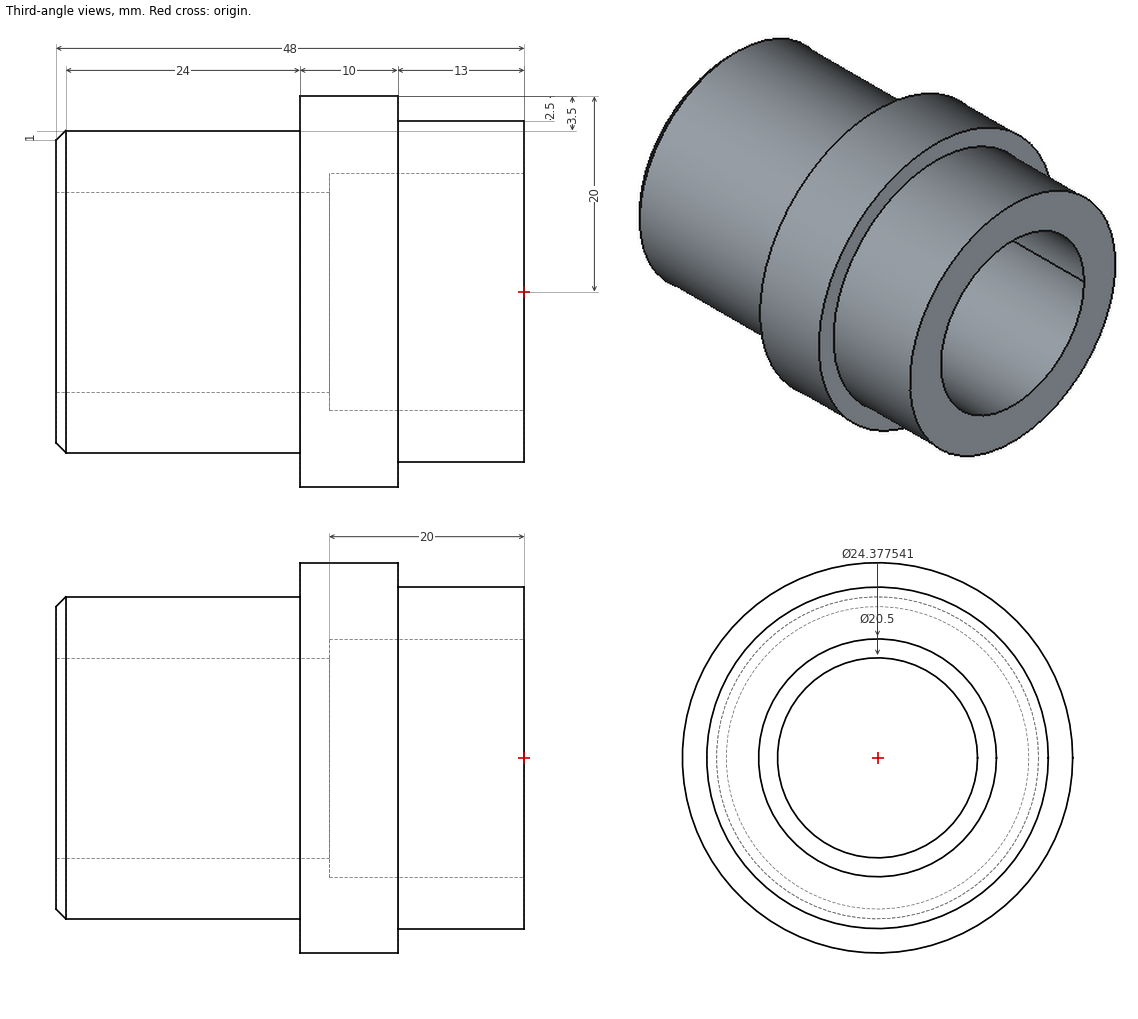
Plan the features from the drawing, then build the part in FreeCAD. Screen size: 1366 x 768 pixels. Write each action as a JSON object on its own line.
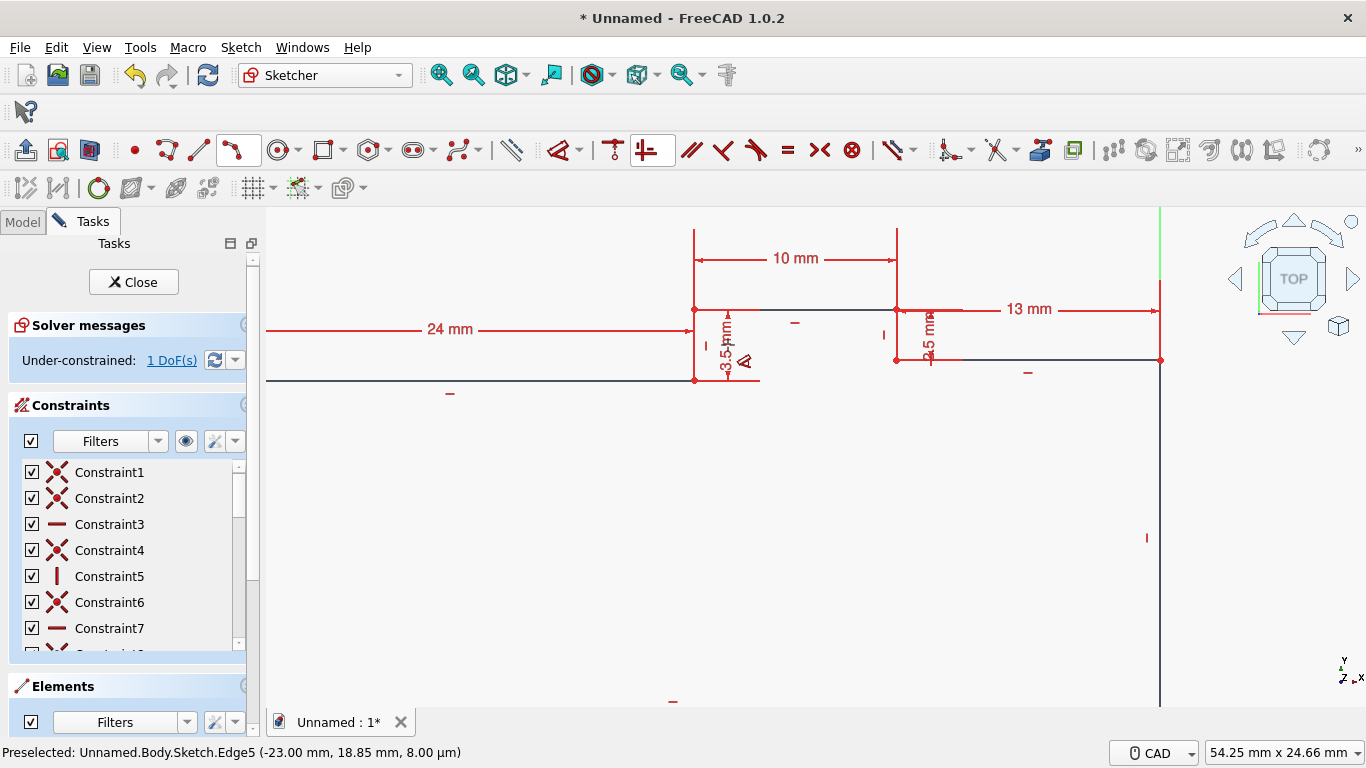
{"action": "left_click", "coordinate": [897, 310]}
{"action": "left_click", "coordinate": [1194, 494]}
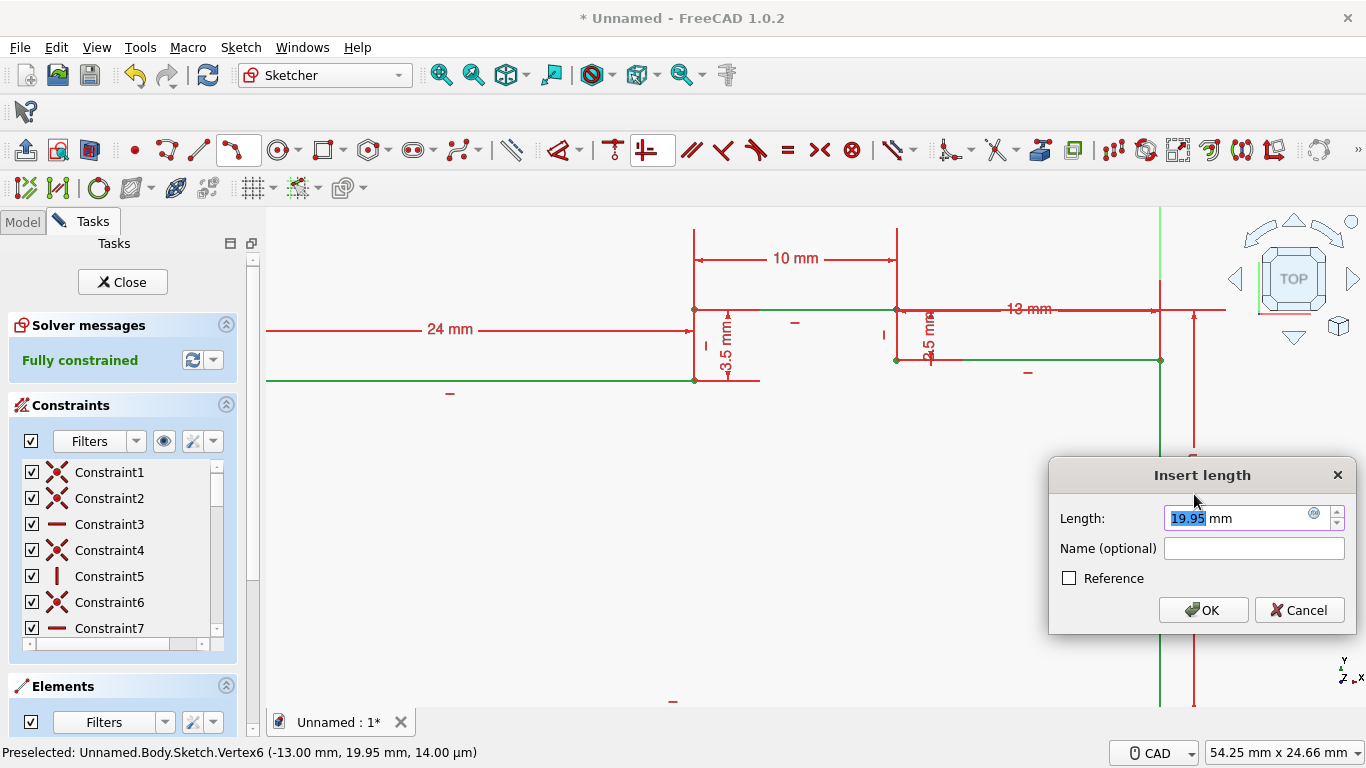
{"action": "type", "text": "20"}
{"action": "key", "text": "Return"}
{"action": "key", "text": "Escape"}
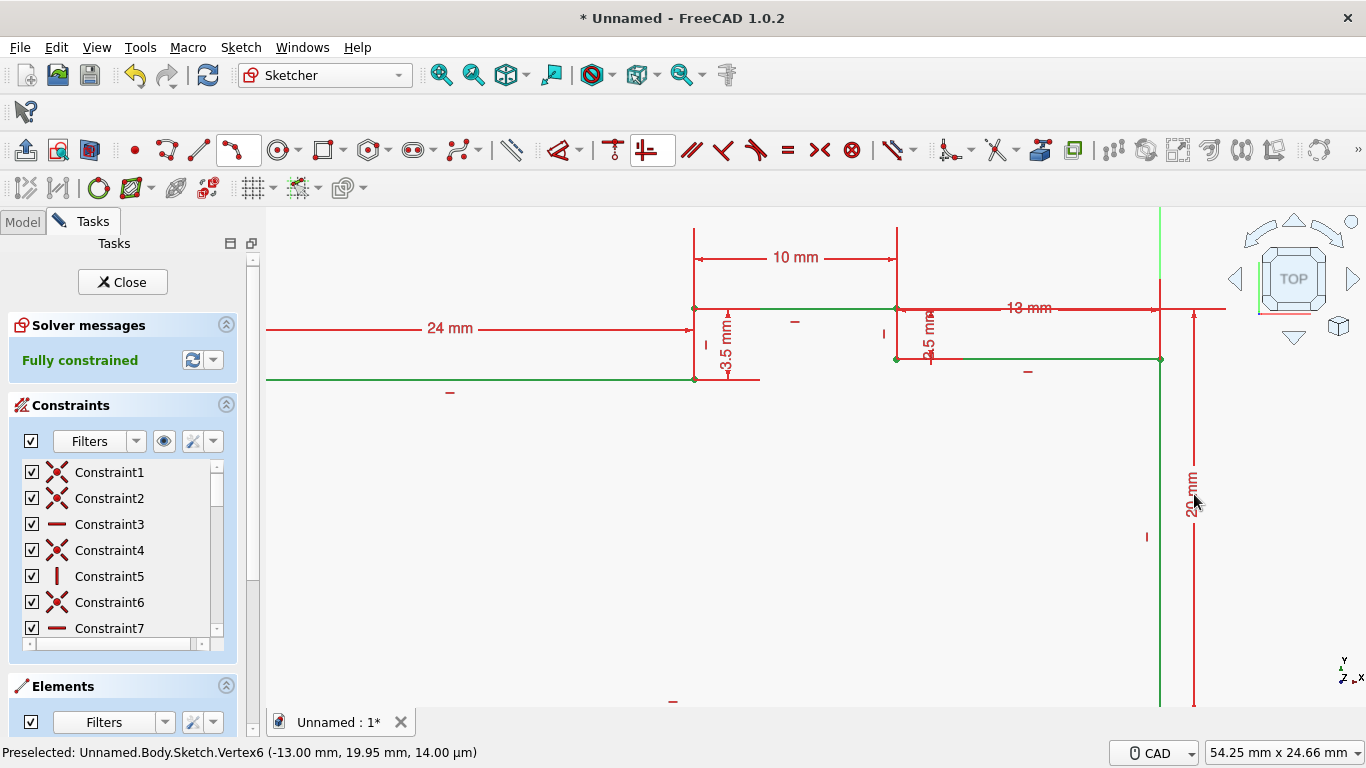
{"action": "left_click", "coordinate": [123, 282]}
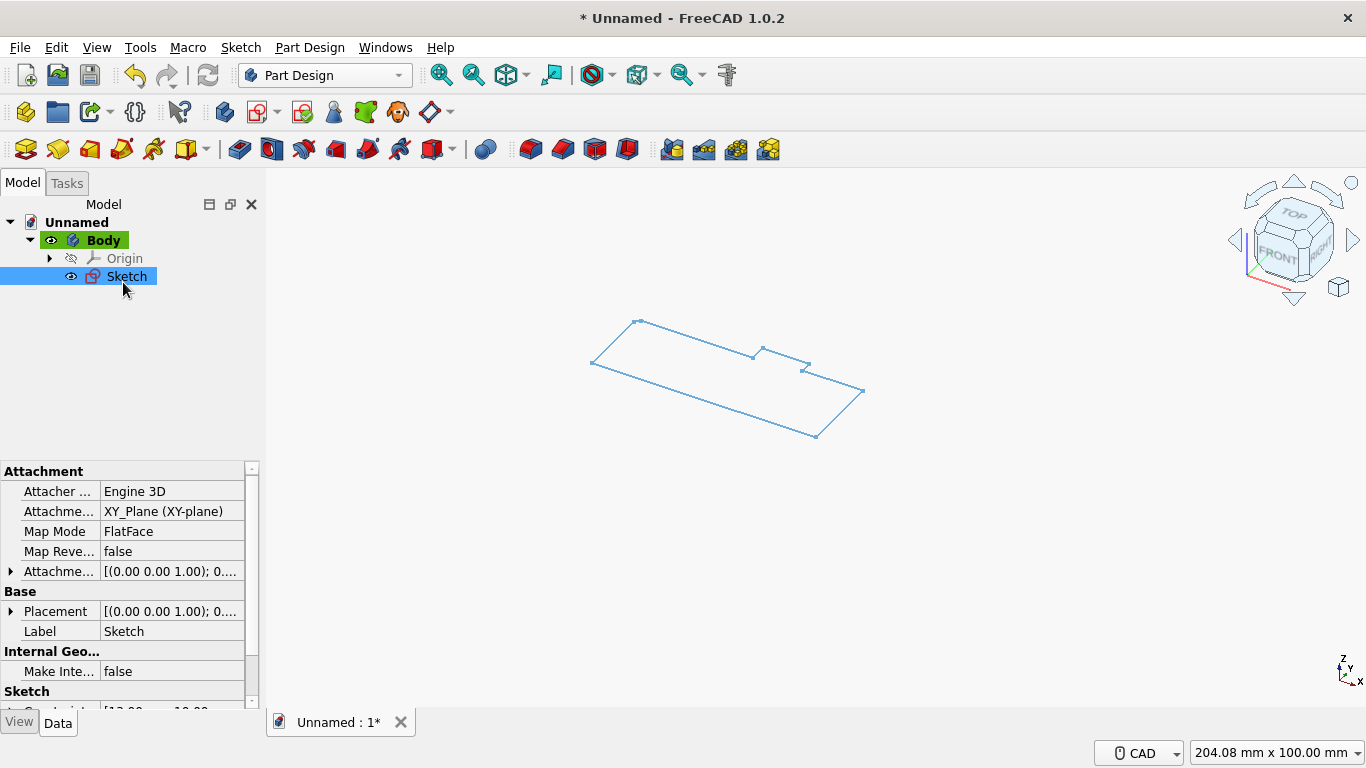
{"action": "left_click", "coordinate": [58, 150]}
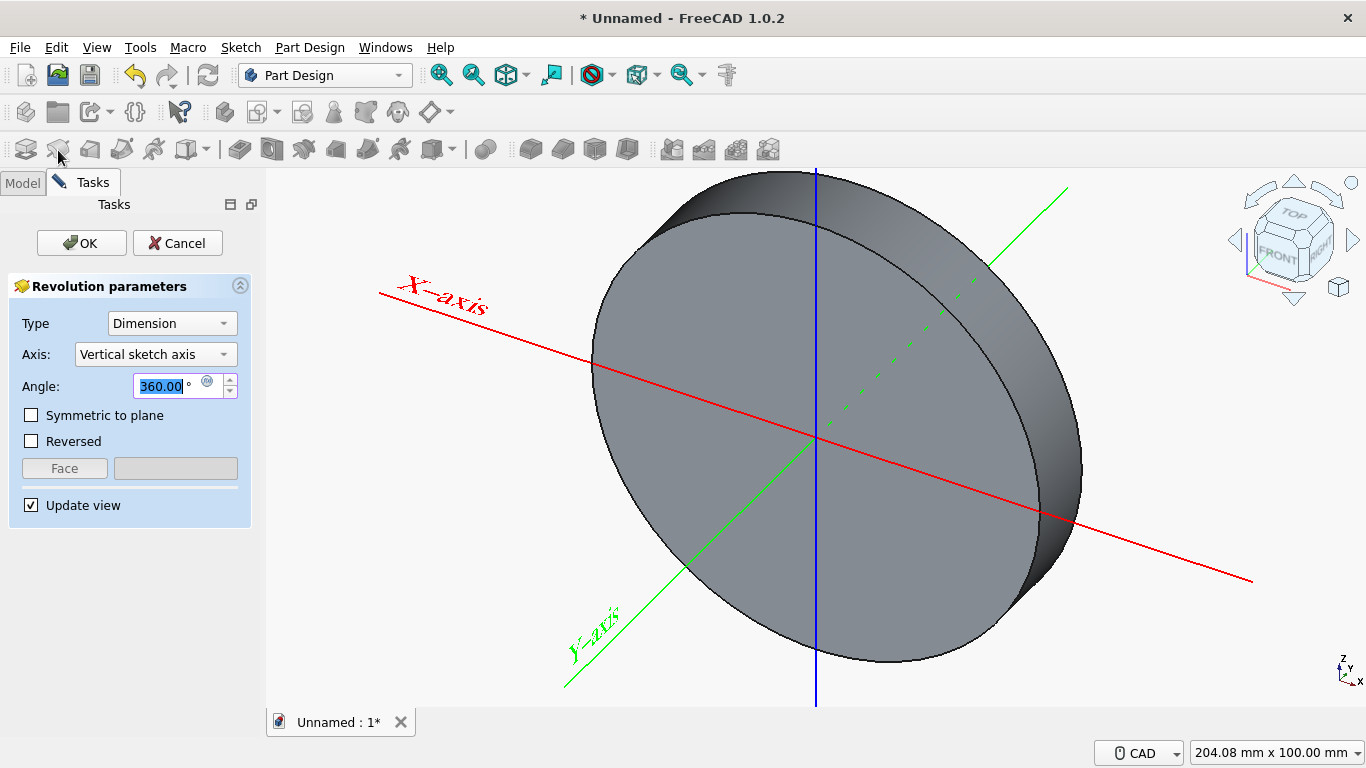
{"action": "left_click", "coordinate": [156, 354]}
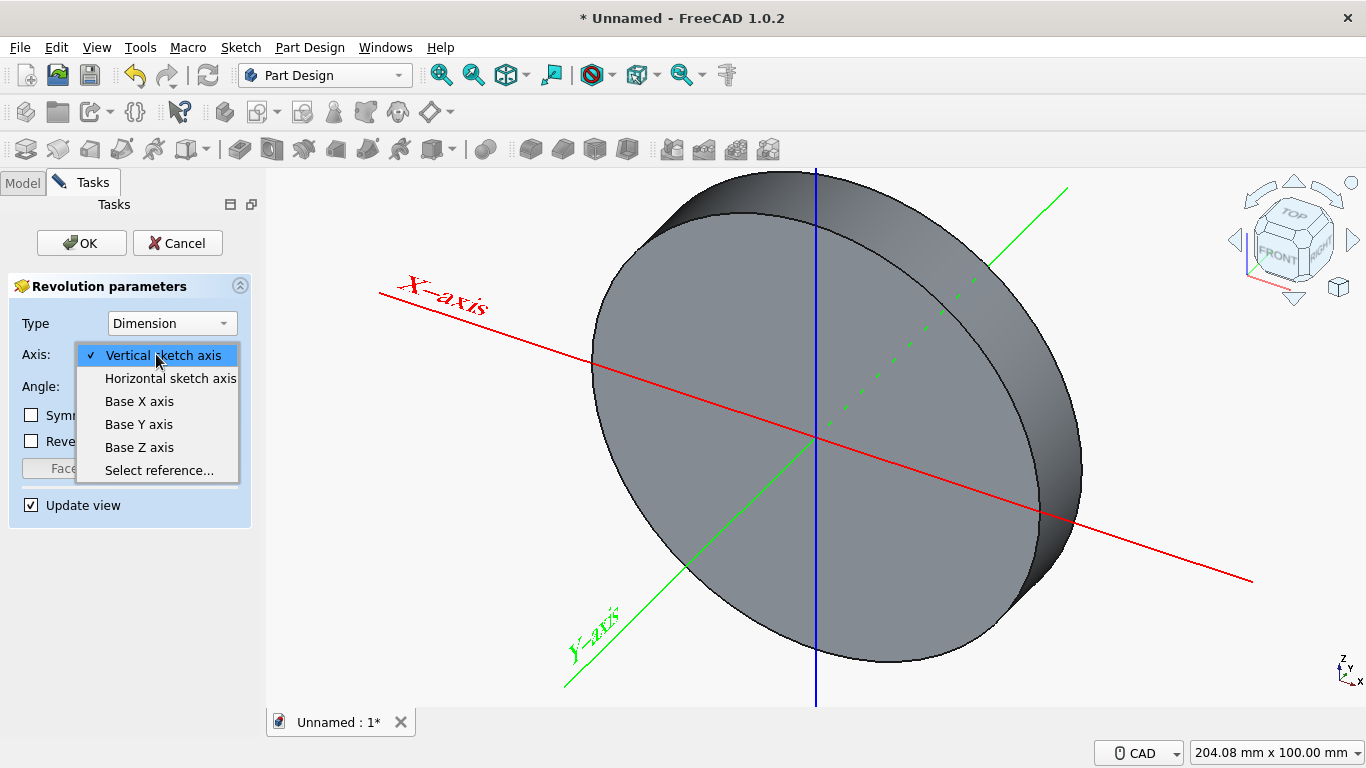
{"action": "left_click", "coordinate": [156, 378]}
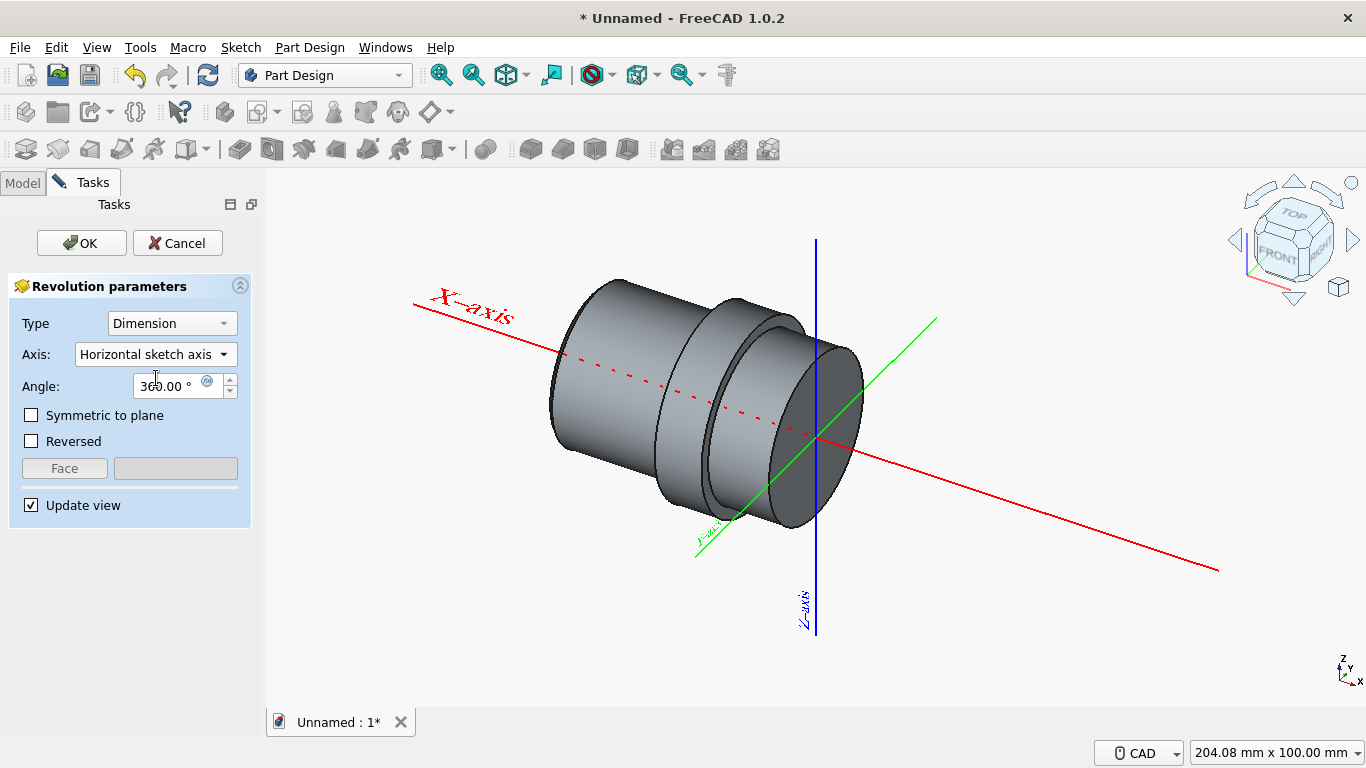
{"action": "left_click", "coordinate": [82, 243]}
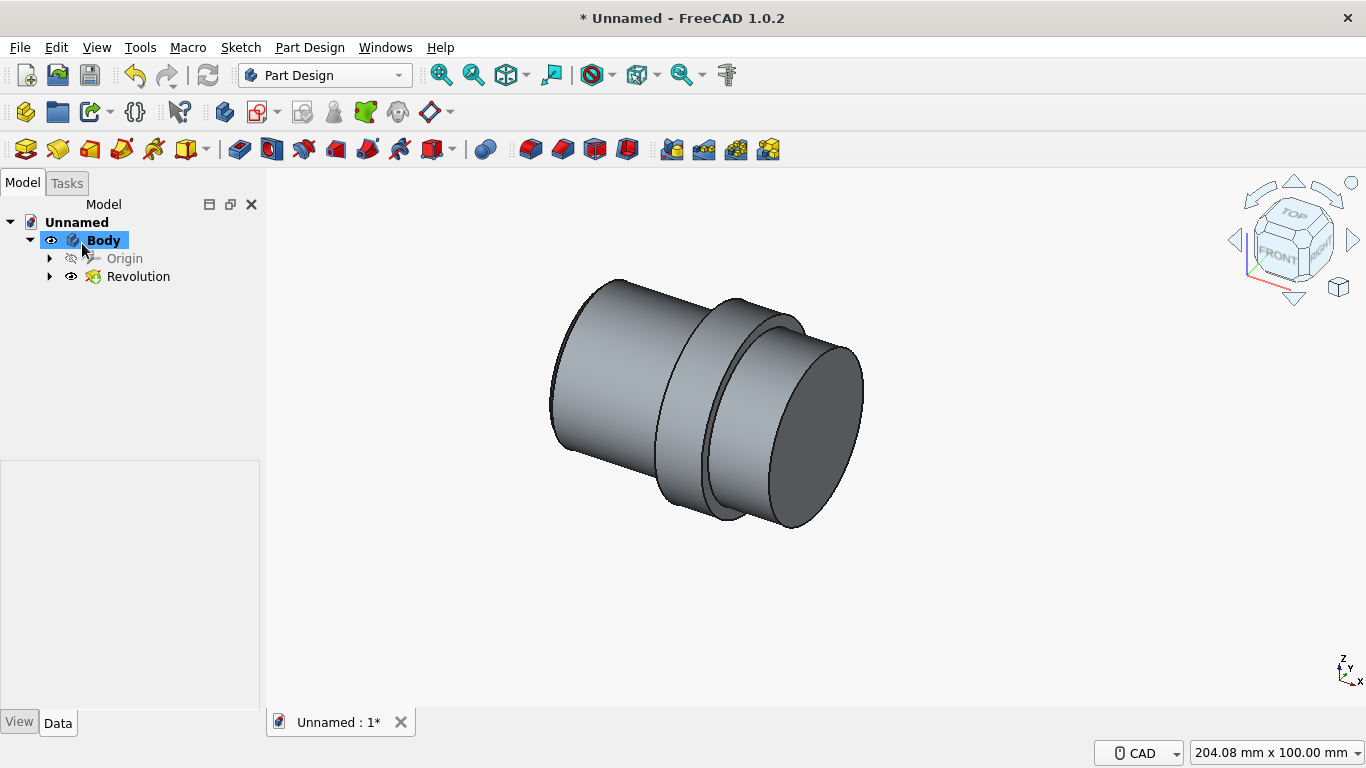
{"action": "left_click", "coordinate": [258, 112]}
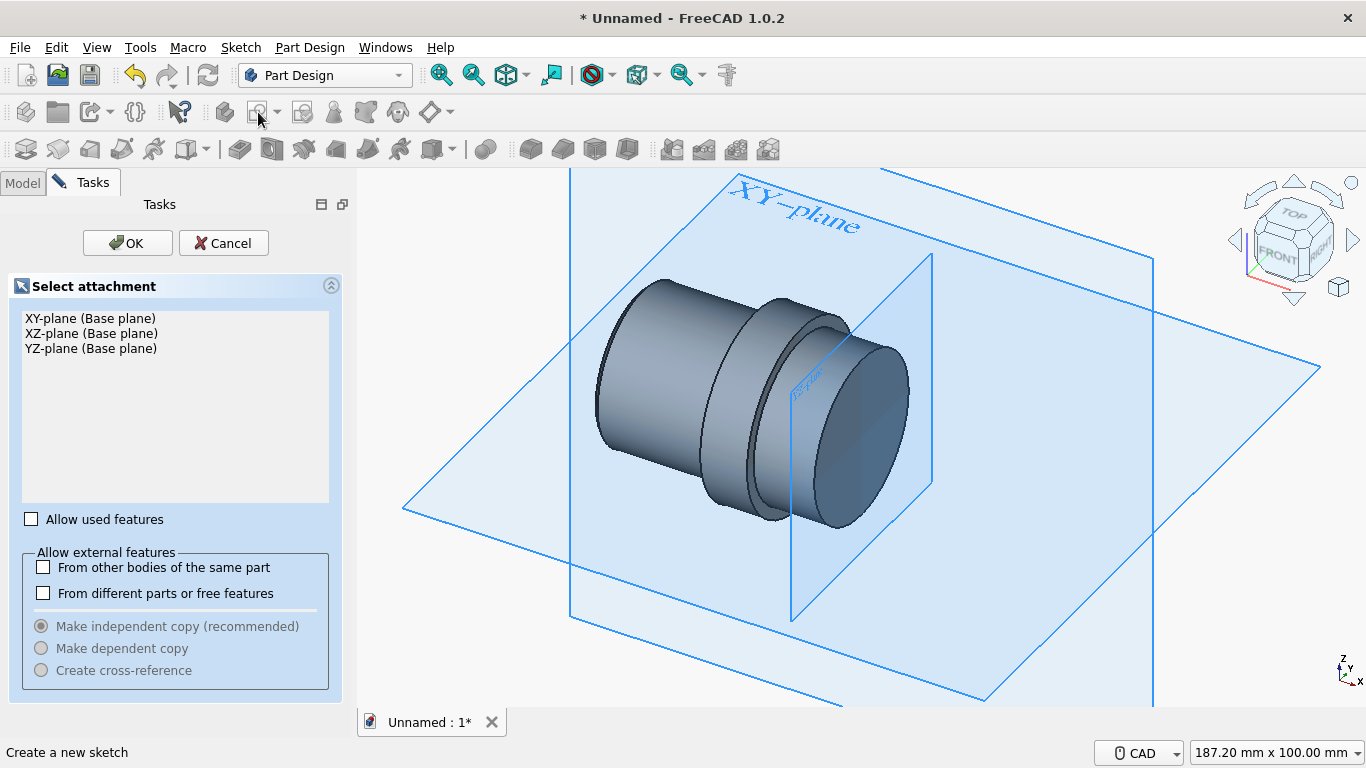
{"action": "left_click", "coordinate": [82, 348]}